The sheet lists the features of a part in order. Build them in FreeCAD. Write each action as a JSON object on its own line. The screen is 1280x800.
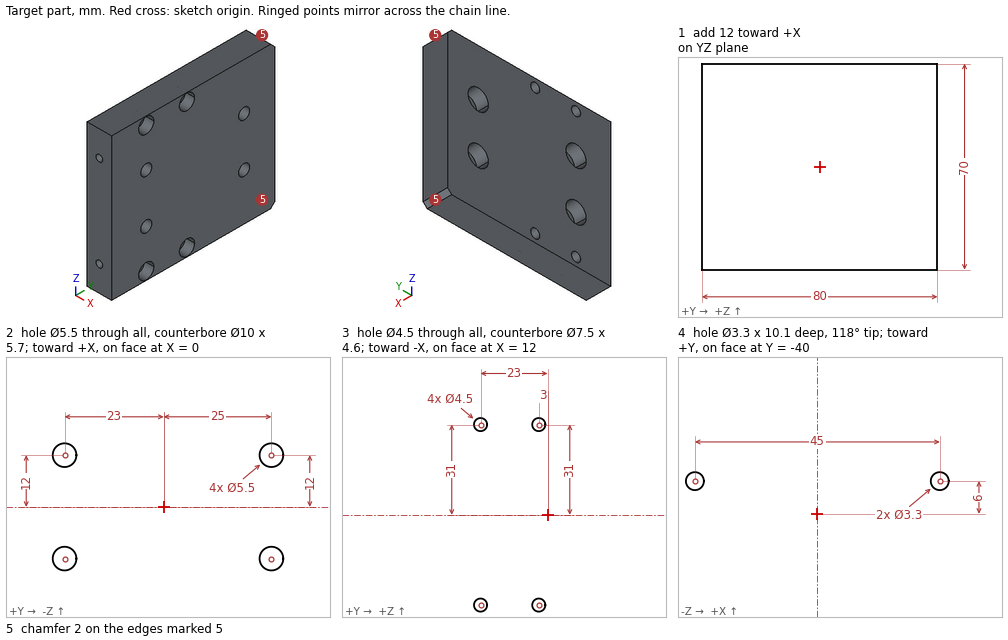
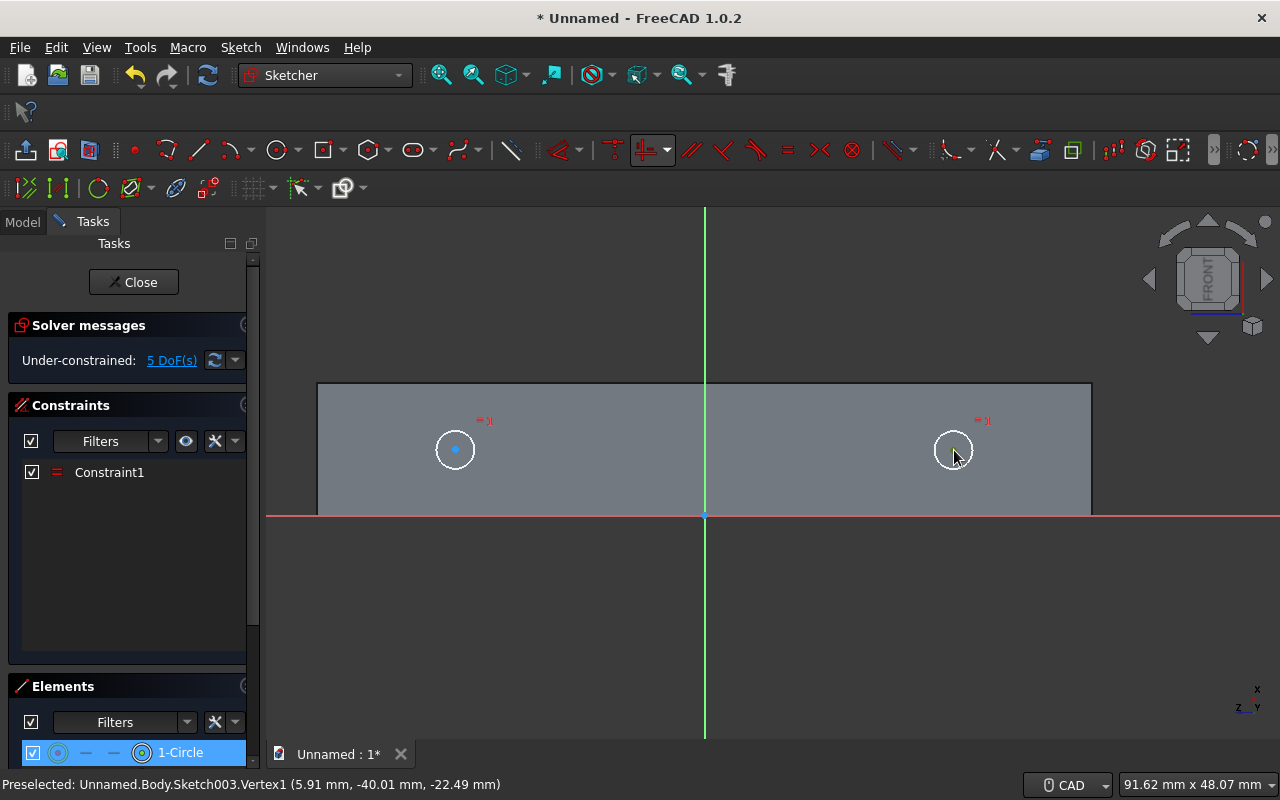
{"action": "left_click", "coordinate": [455, 450]}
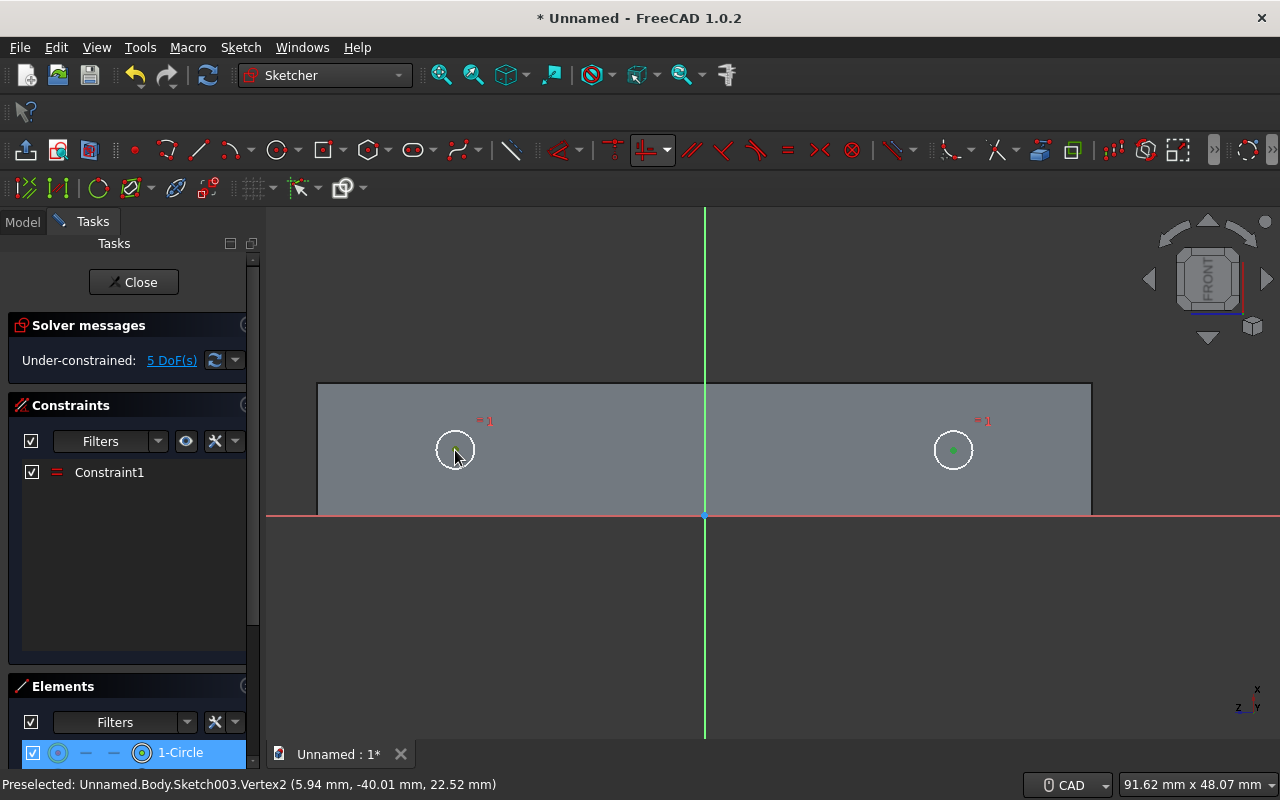
{"action": "left_click", "coordinate": [705, 677]}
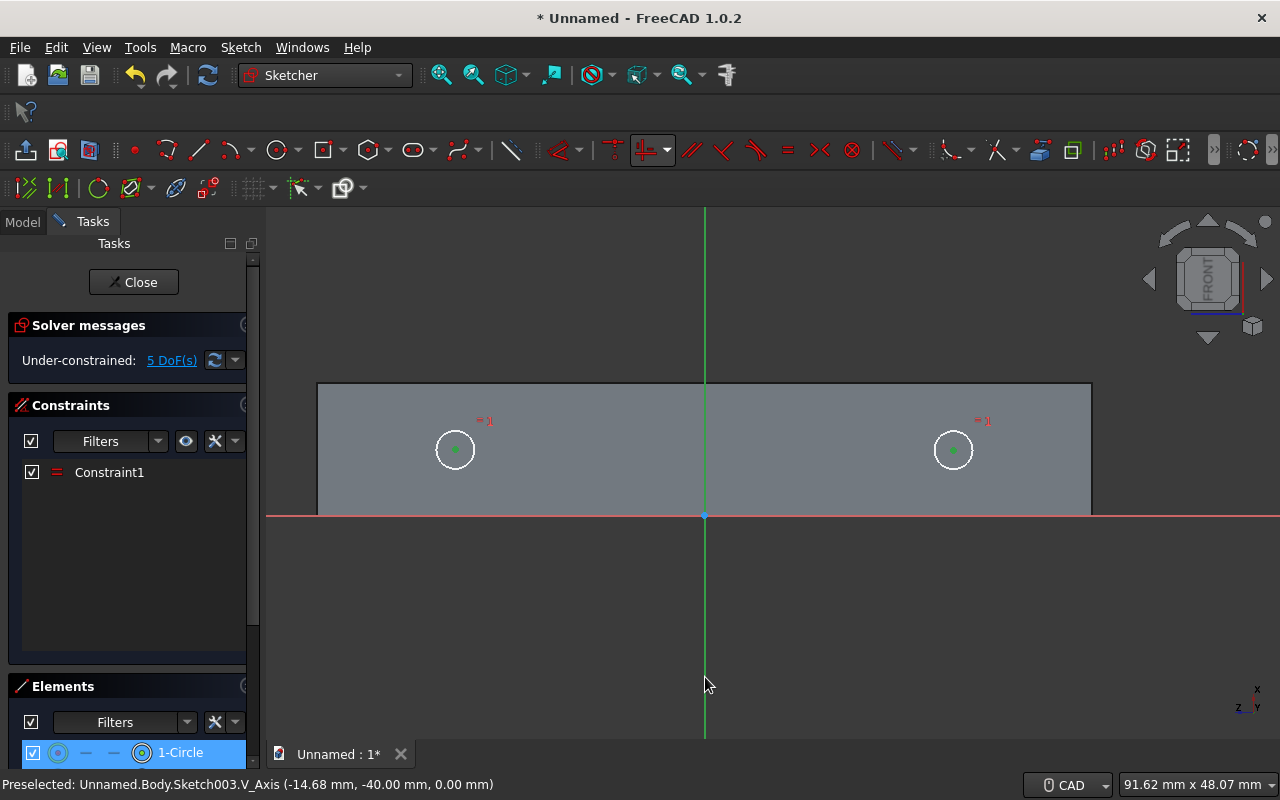
{"action": "left_click", "coordinate": [820, 150]}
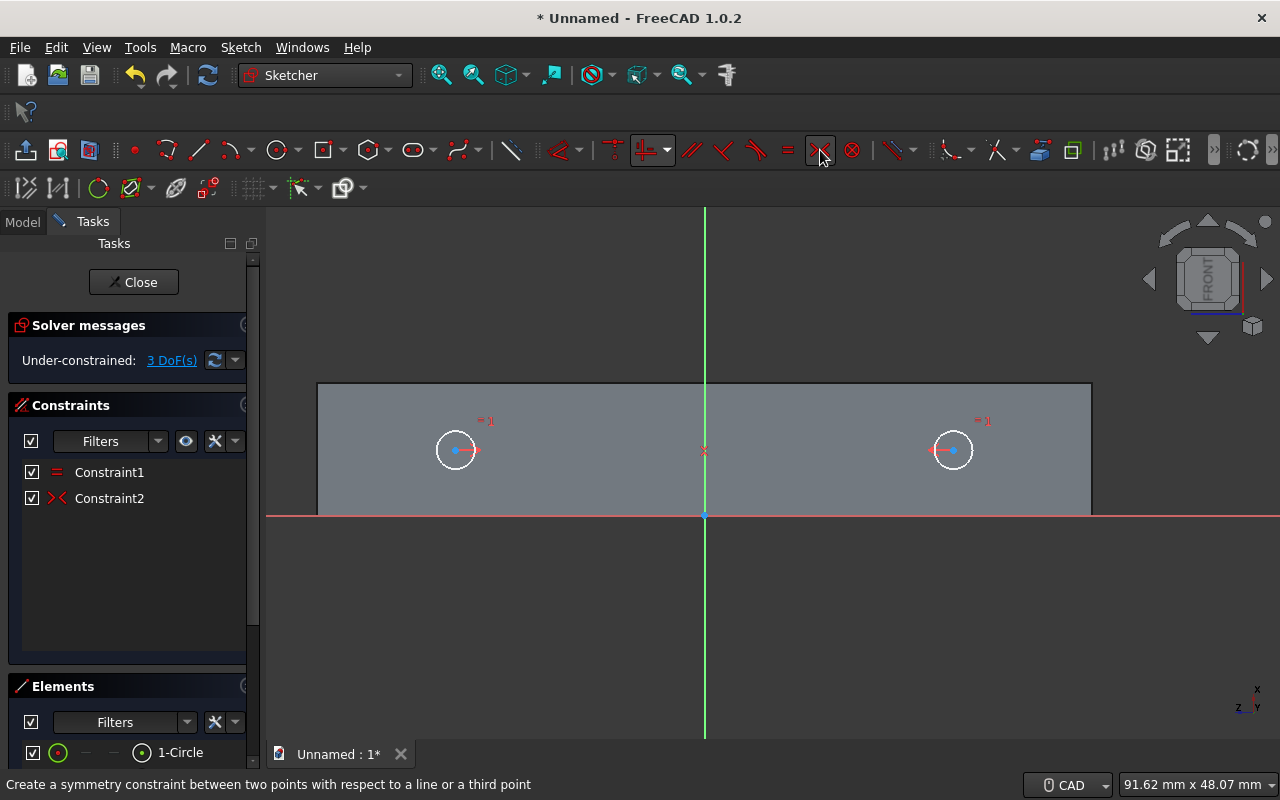
{"action": "left_click", "coordinate": [558, 150]}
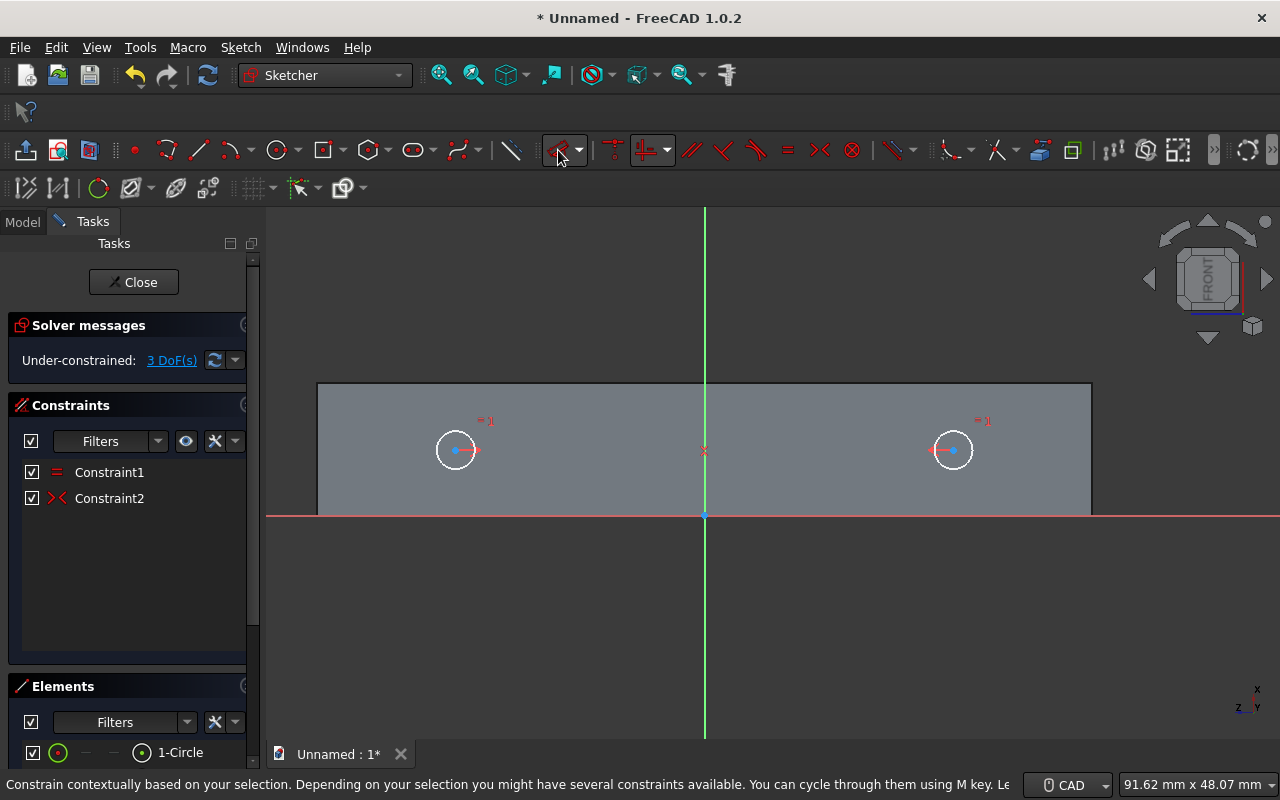
{"action": "left_click", "coordinate": [967, 437]}
{"action": "left_click", "coordinate": [990, 415]}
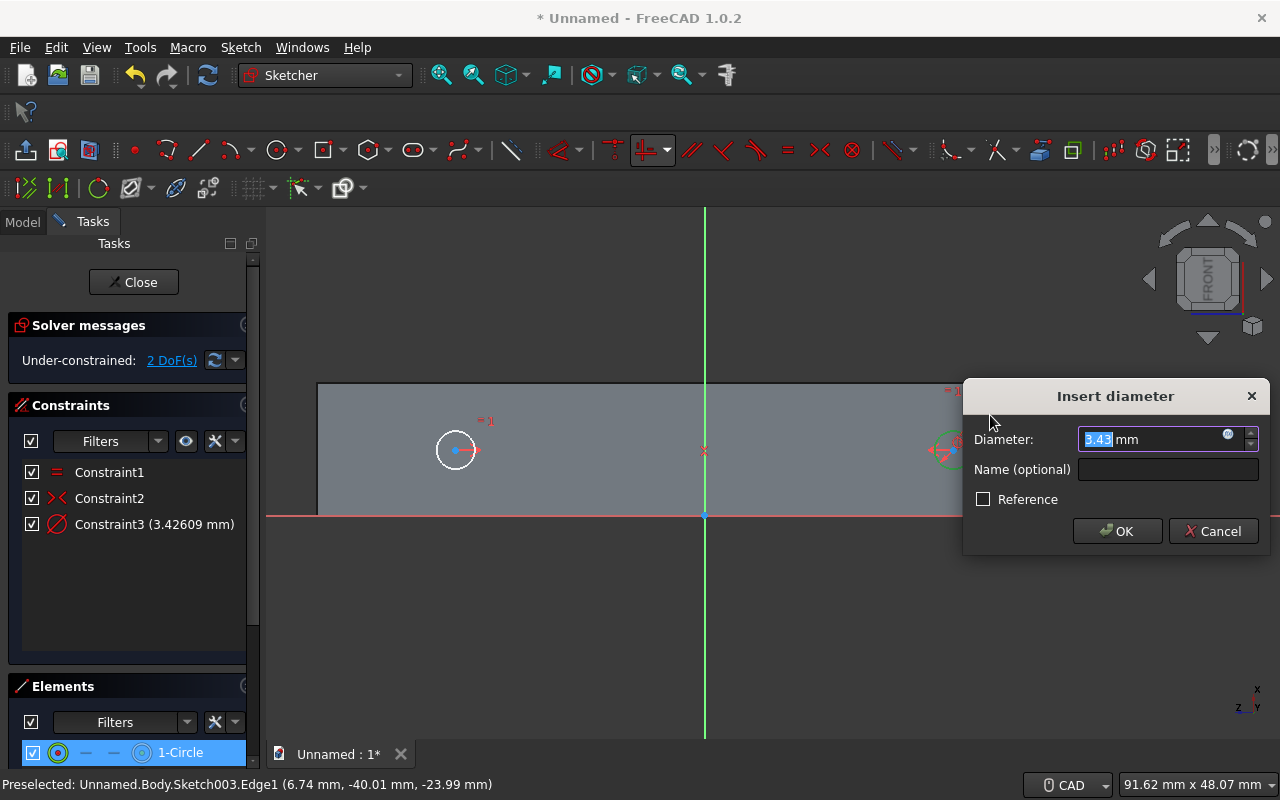
{"action": "type", "text": "3.3"}
{"action": "key", "text": "Return"}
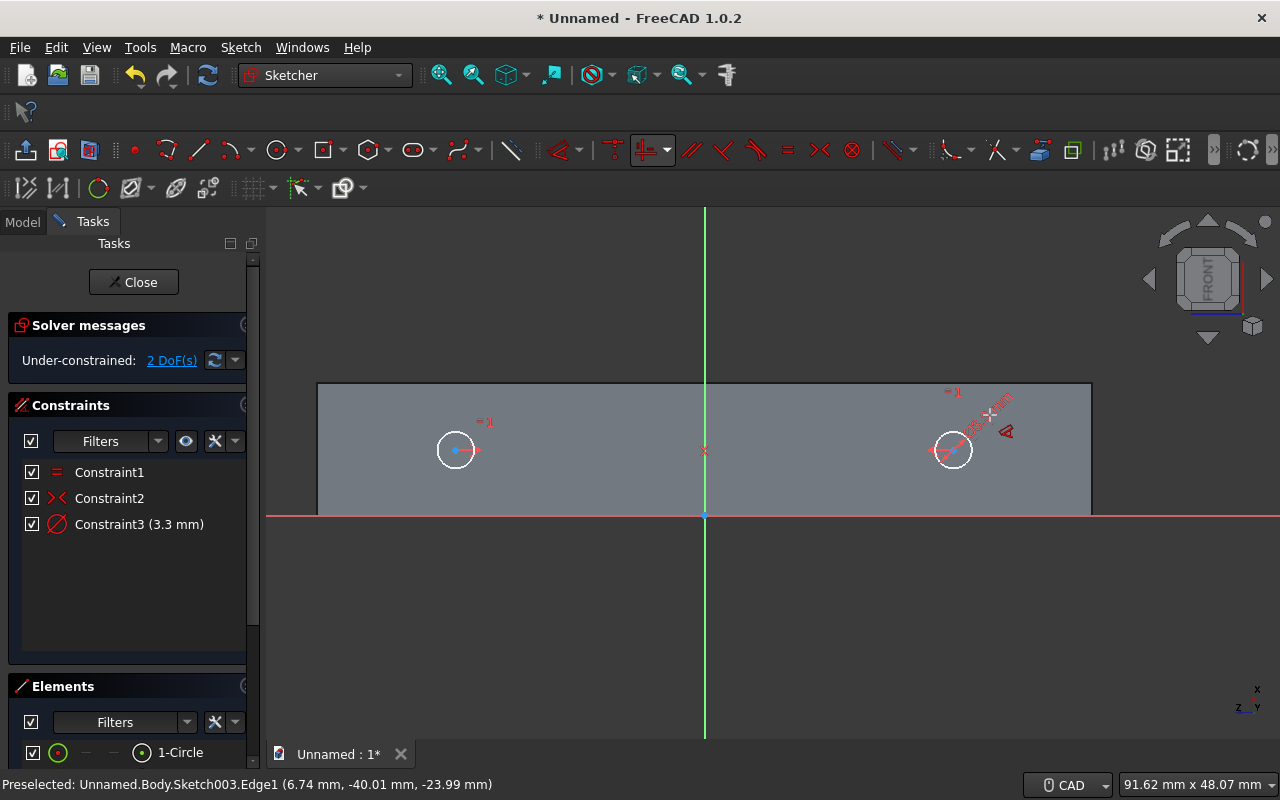
{"action": "left_click", "coordinate": [954, 450]}
{"action": "left_click", "coordinate": [988, 483]}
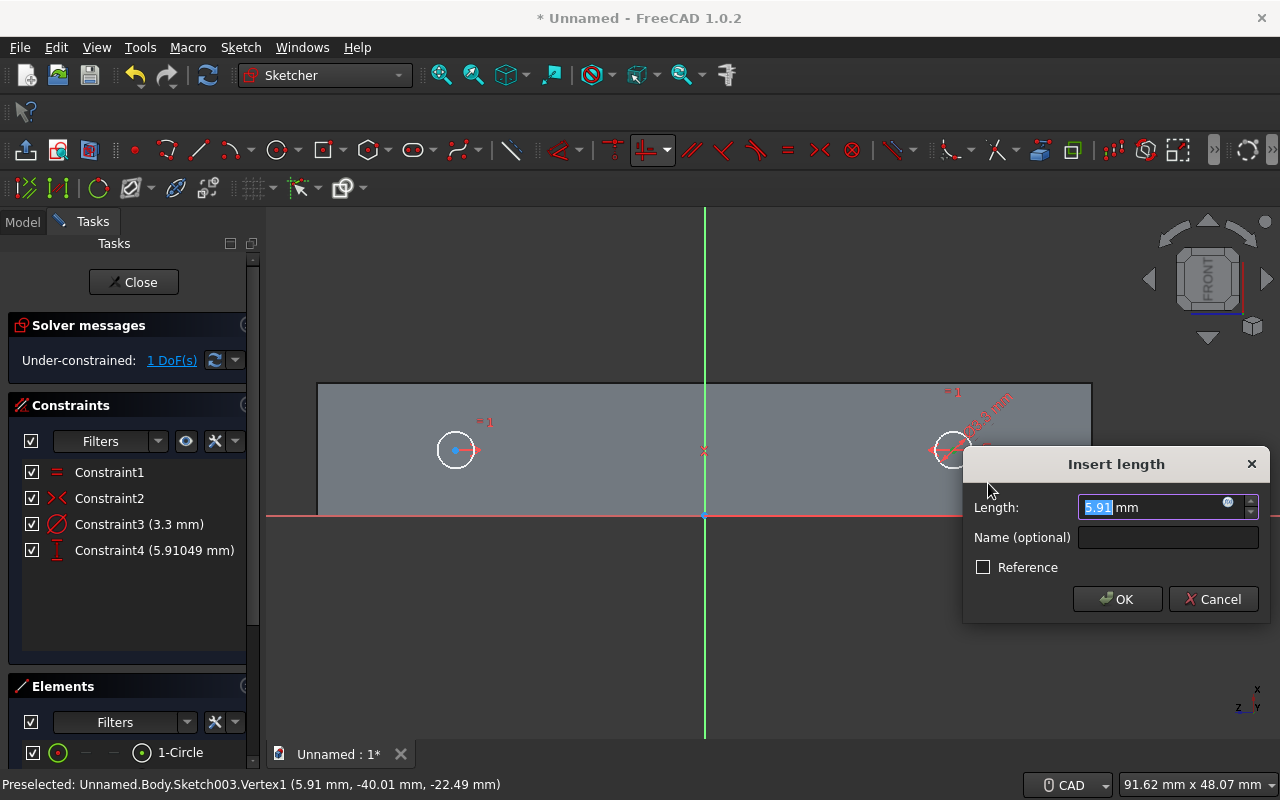
{"action": "type", "text": "6"}
{"action": "key", "text": "Return"}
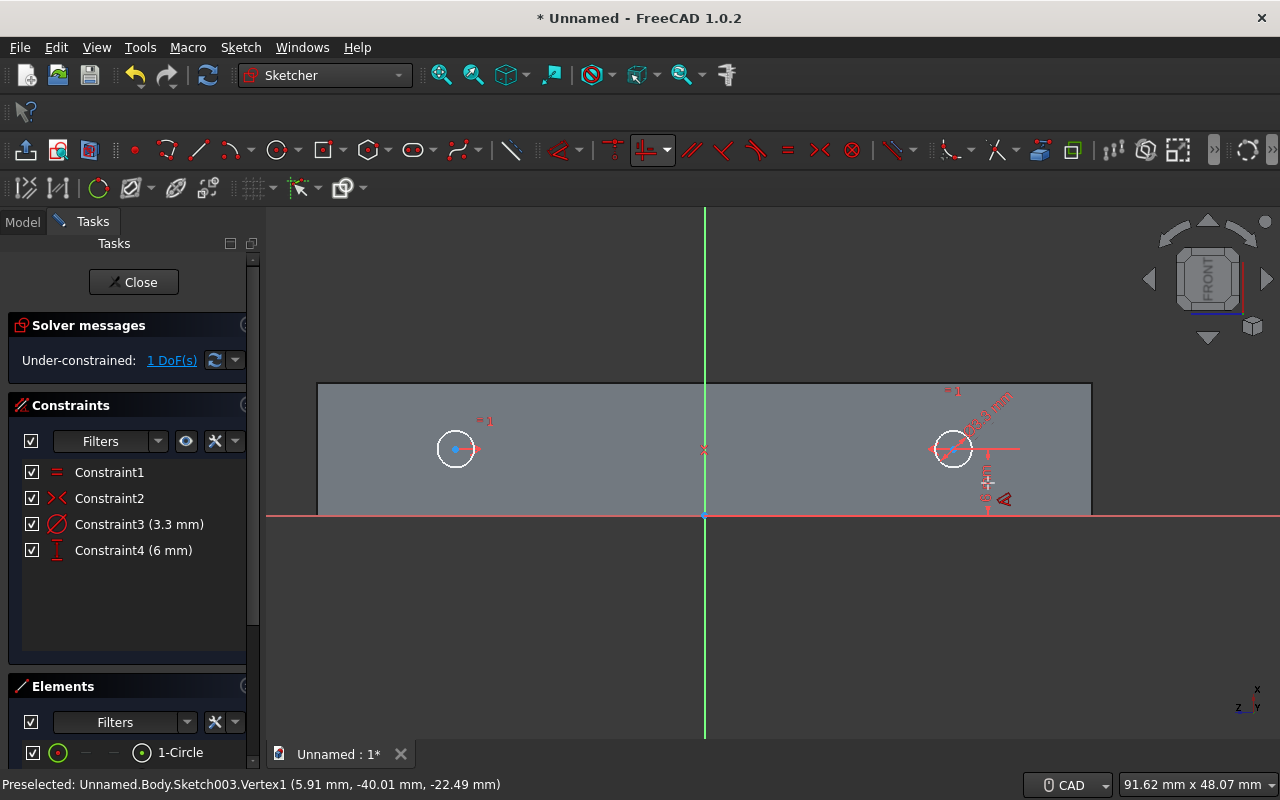
{"action": "left_click", "coordinate": [954, 449]}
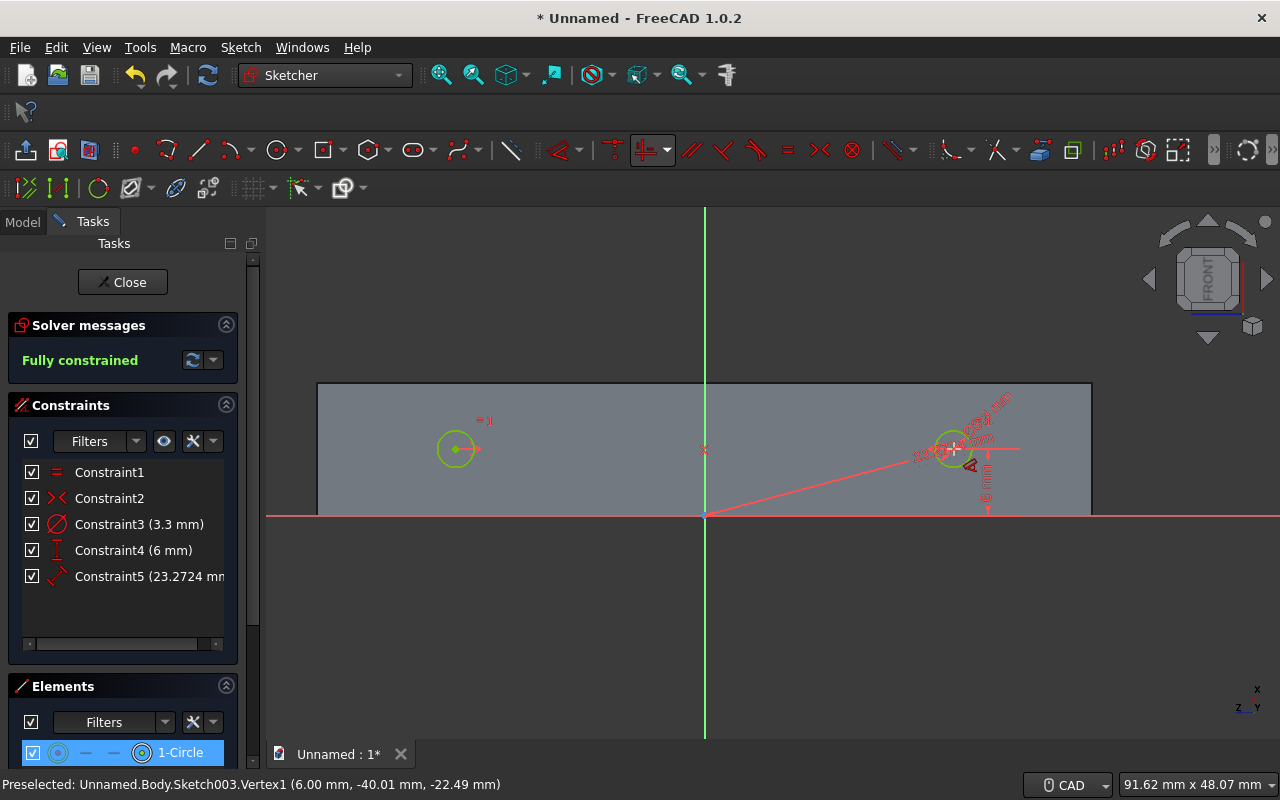
{"action": "left_click", "coordinate": [456, 449]}
{"action": "left_click", "coordinate": [590, 415]}